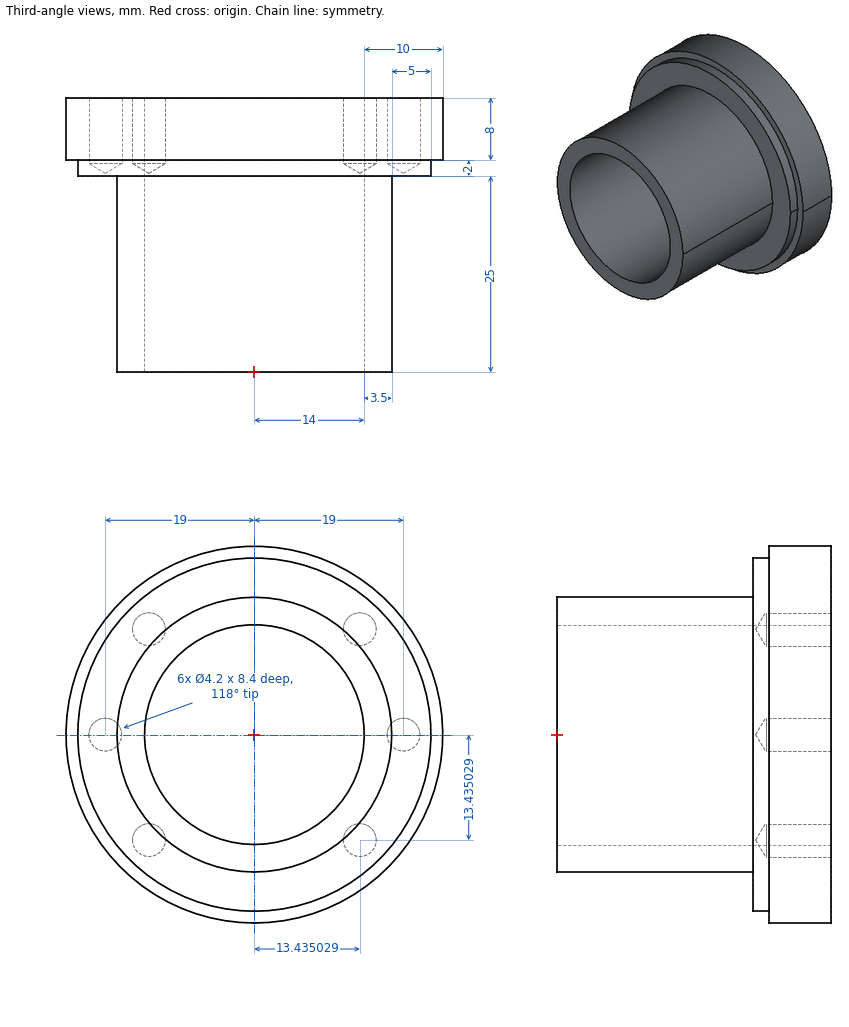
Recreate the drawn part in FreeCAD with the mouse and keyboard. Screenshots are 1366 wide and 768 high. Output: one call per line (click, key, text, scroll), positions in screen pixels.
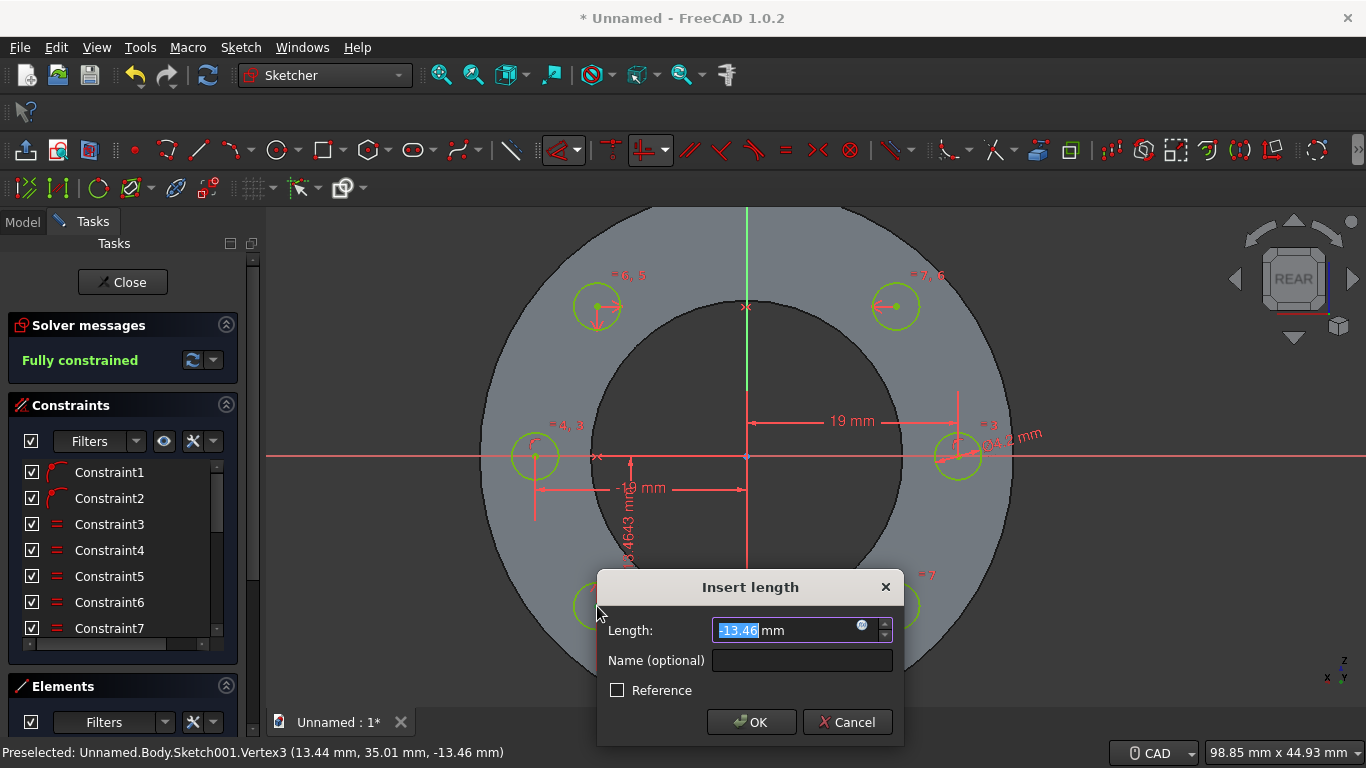
text(-13.435029)
key(Return)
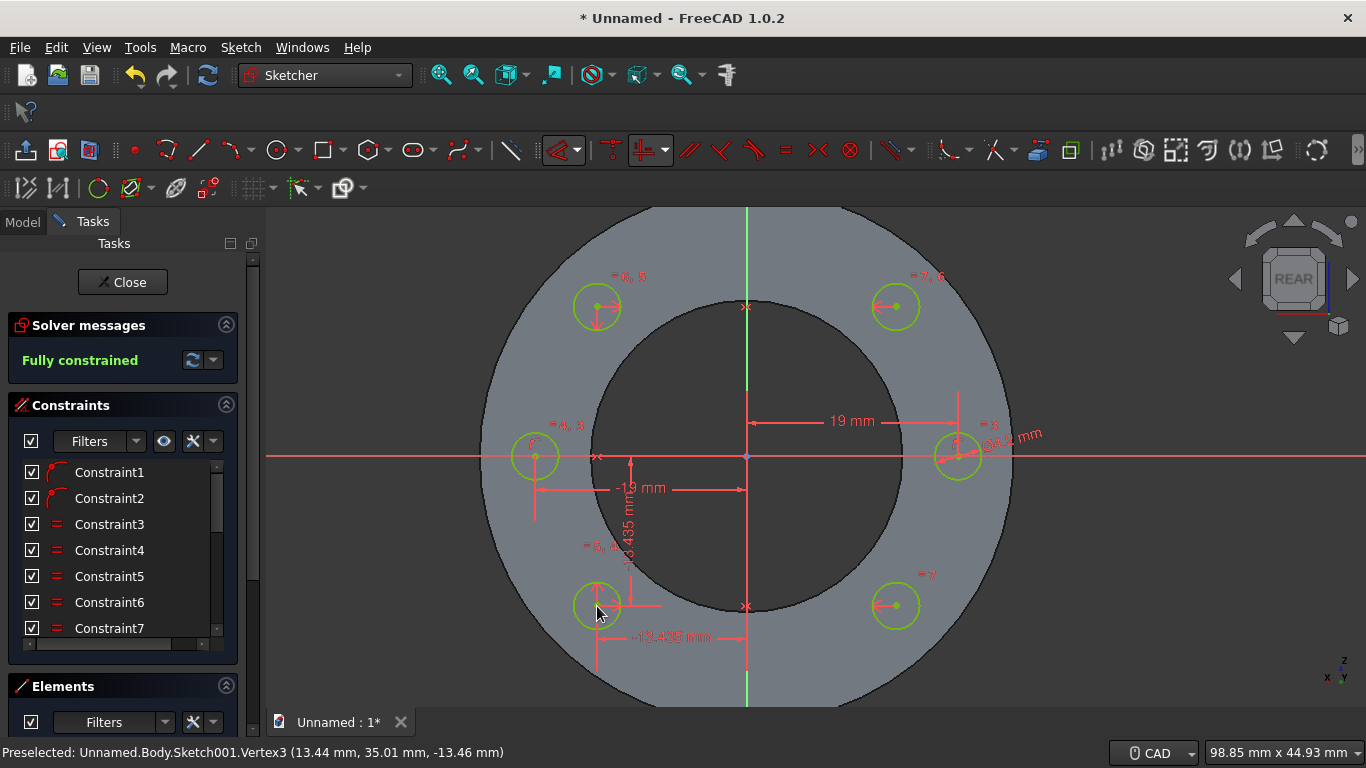
click(123, 282)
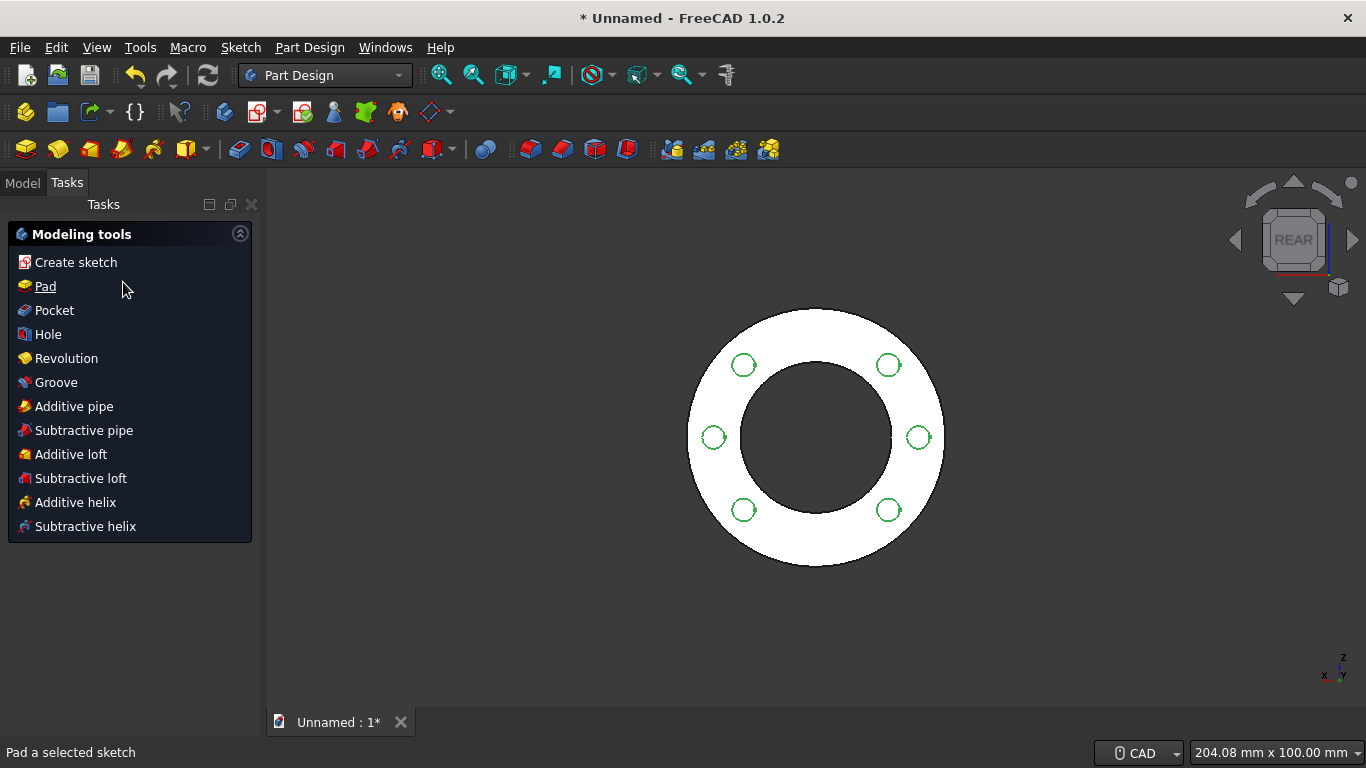
click(272, 150)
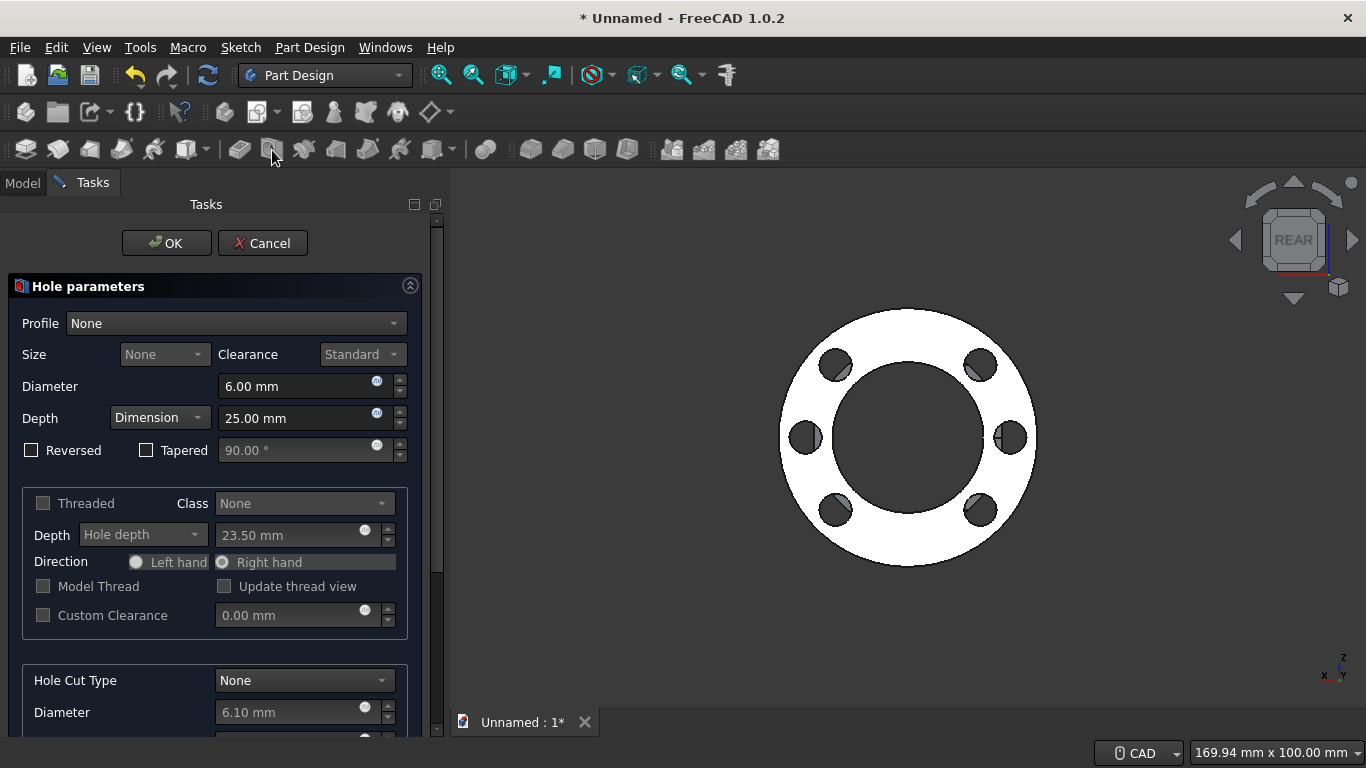
triple_click(305, 386)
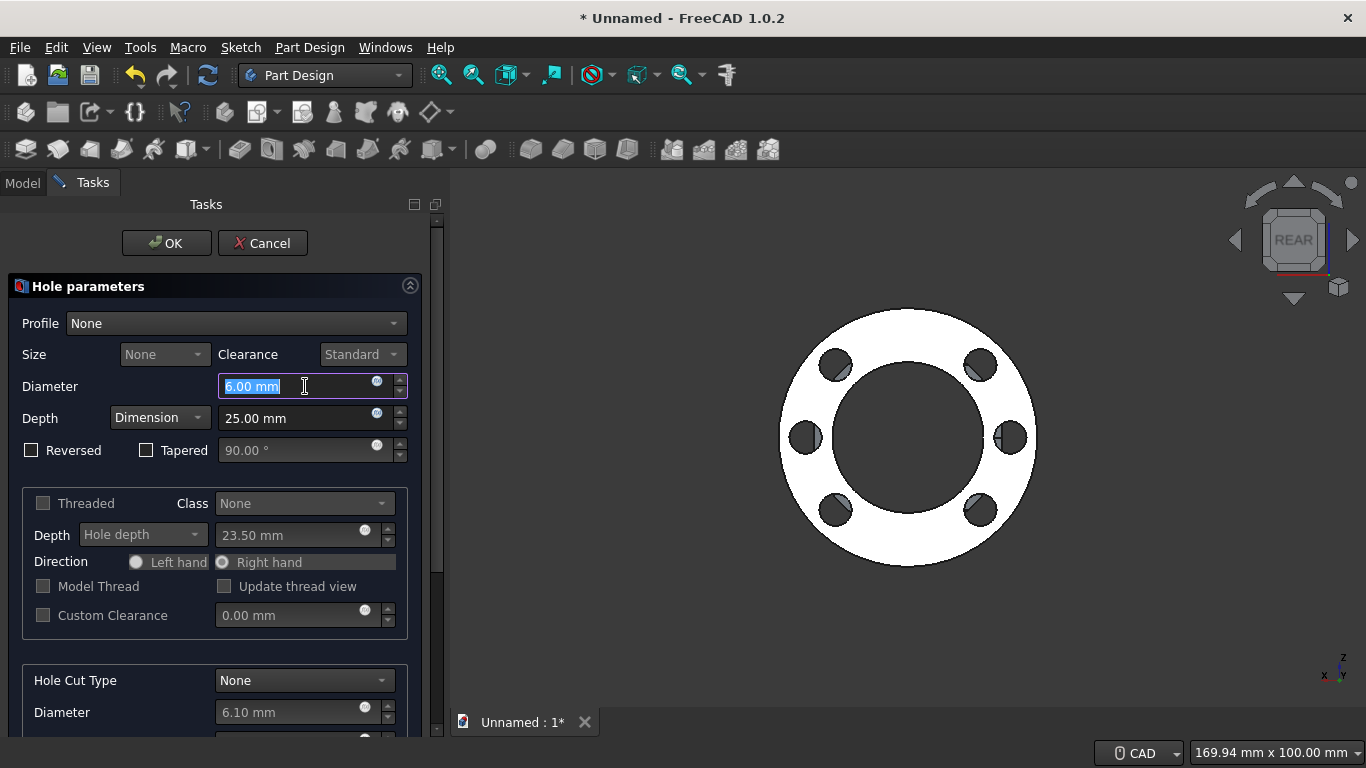
text(4.2)
key(Tab)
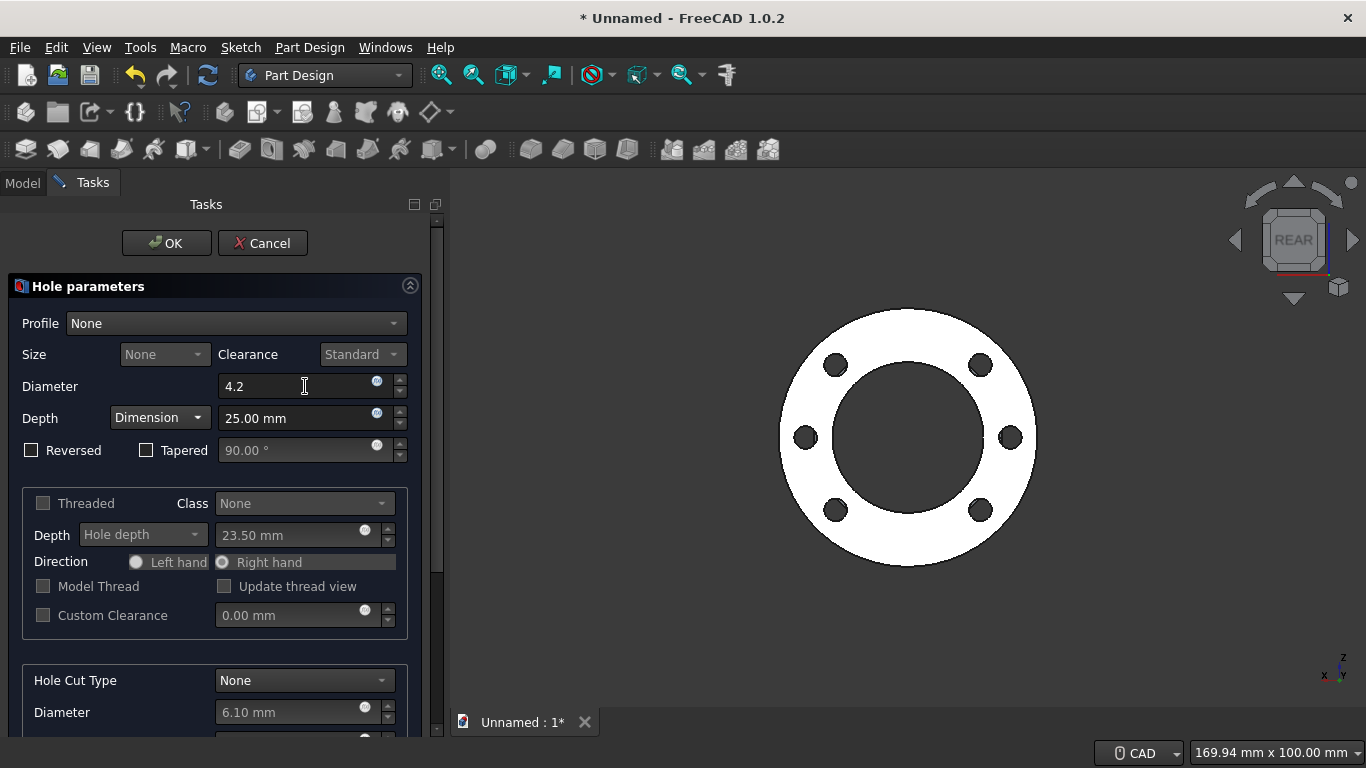
triple_click(305, 418)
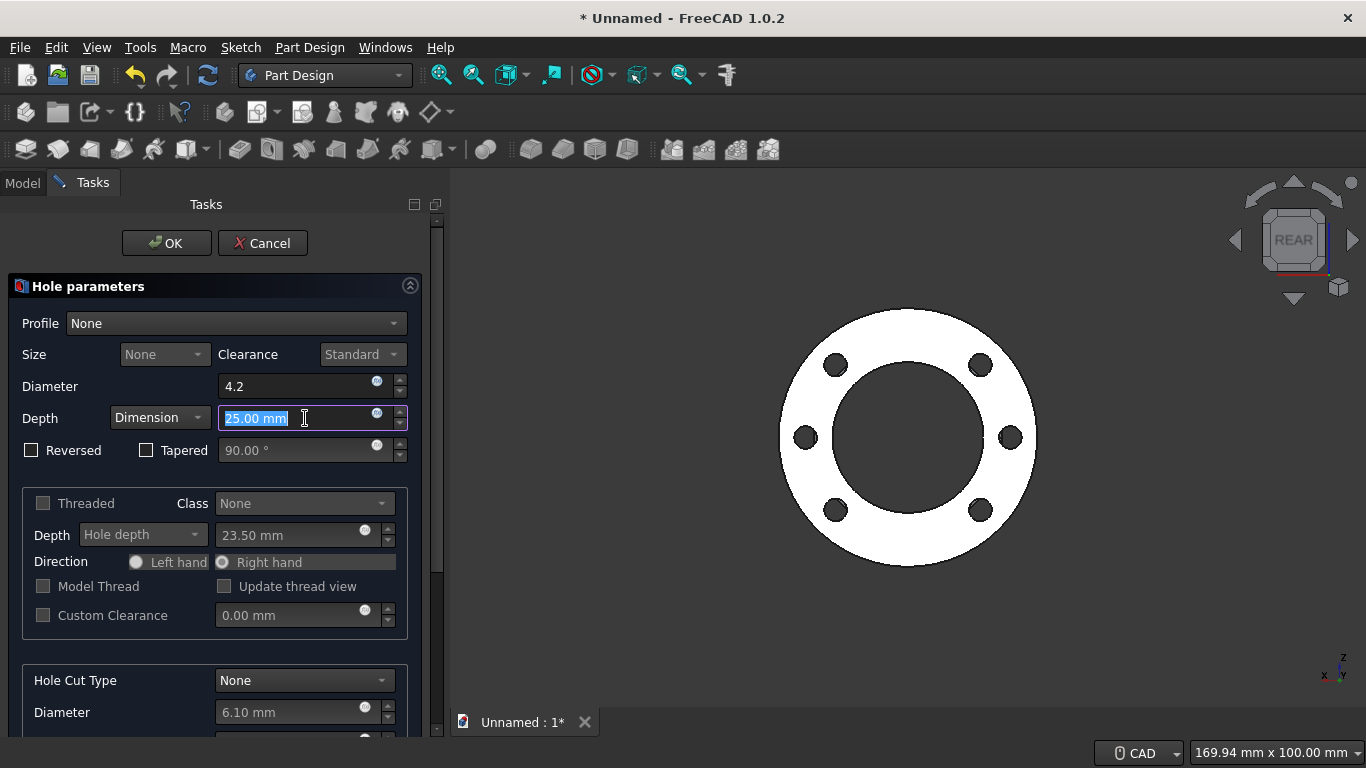
text(8.4)
key(Tab)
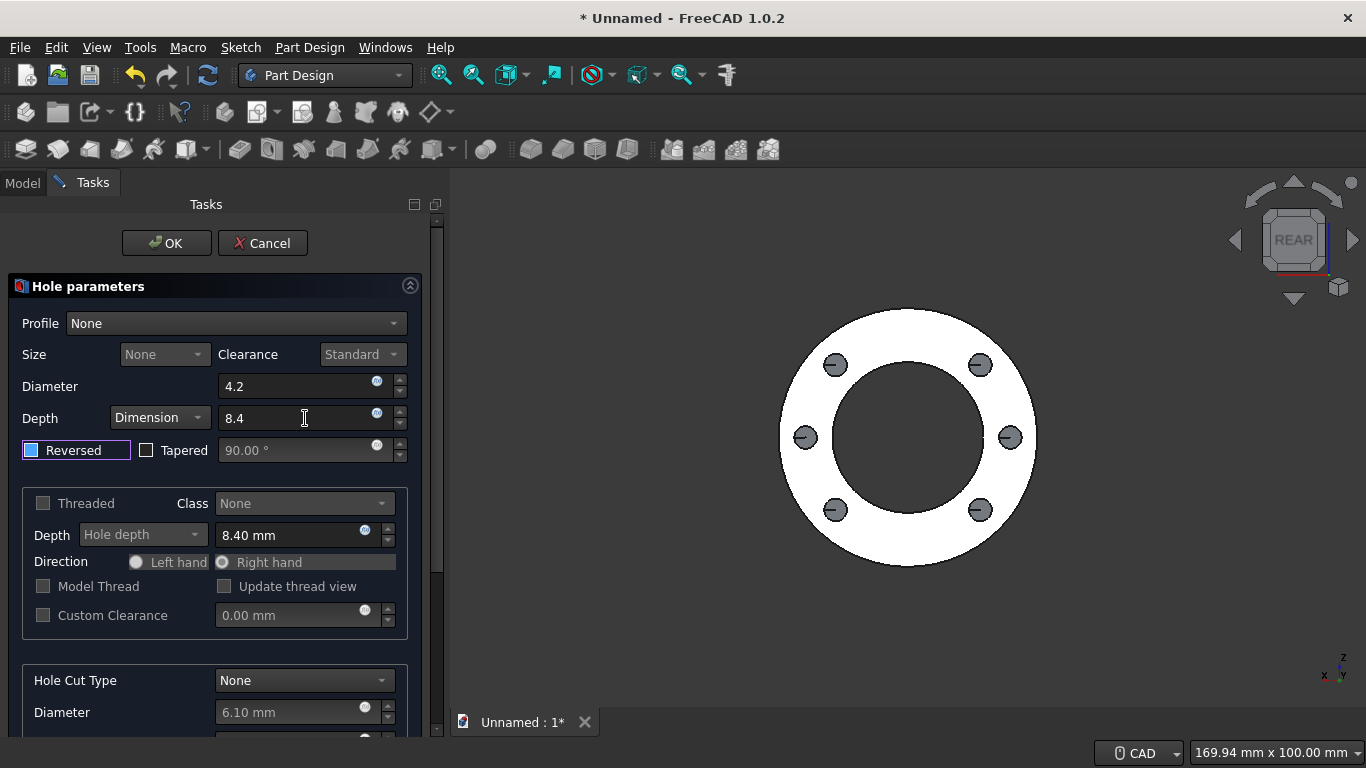
click(167, 243)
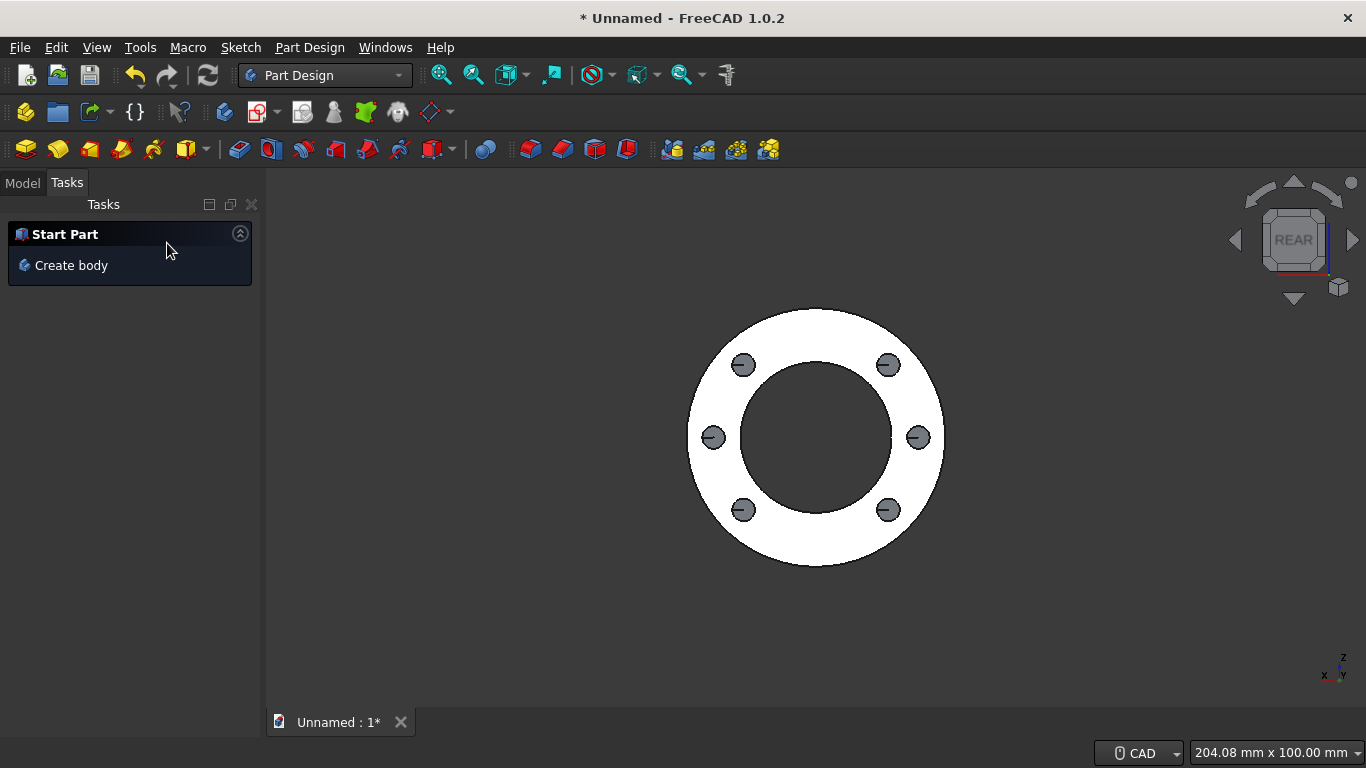
key(0)